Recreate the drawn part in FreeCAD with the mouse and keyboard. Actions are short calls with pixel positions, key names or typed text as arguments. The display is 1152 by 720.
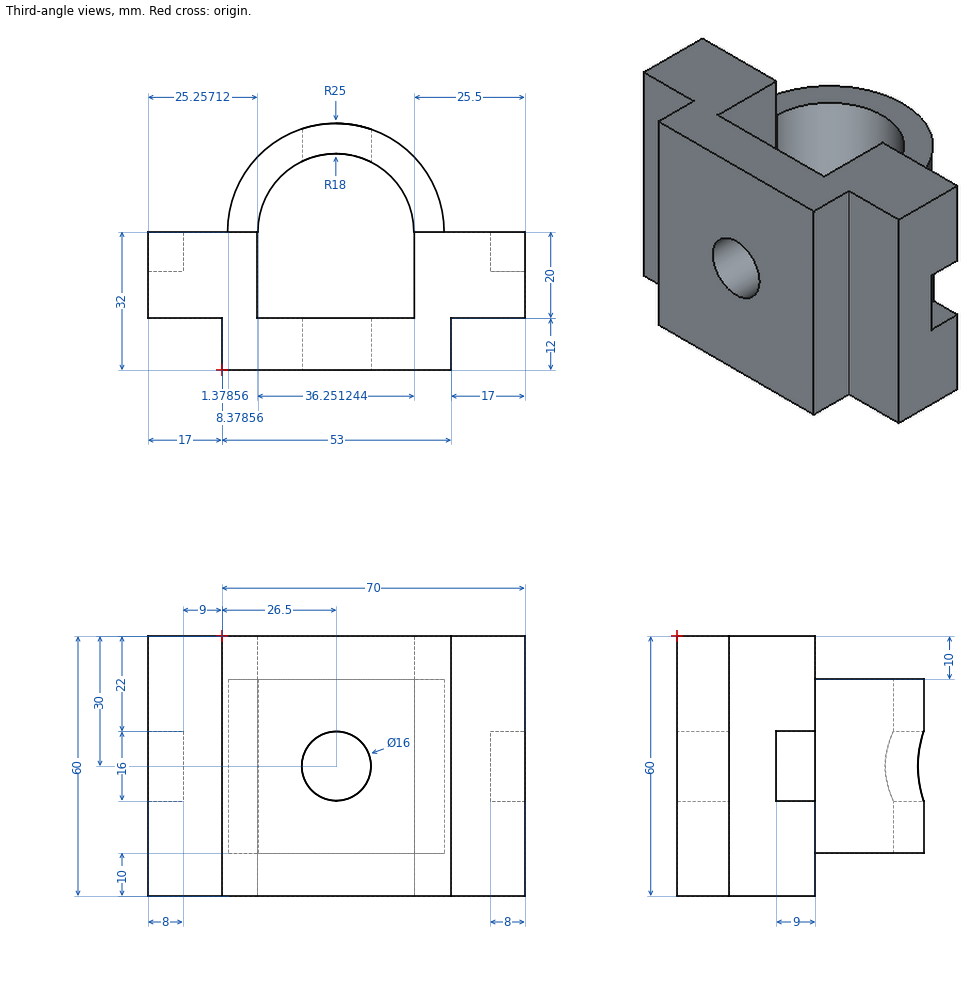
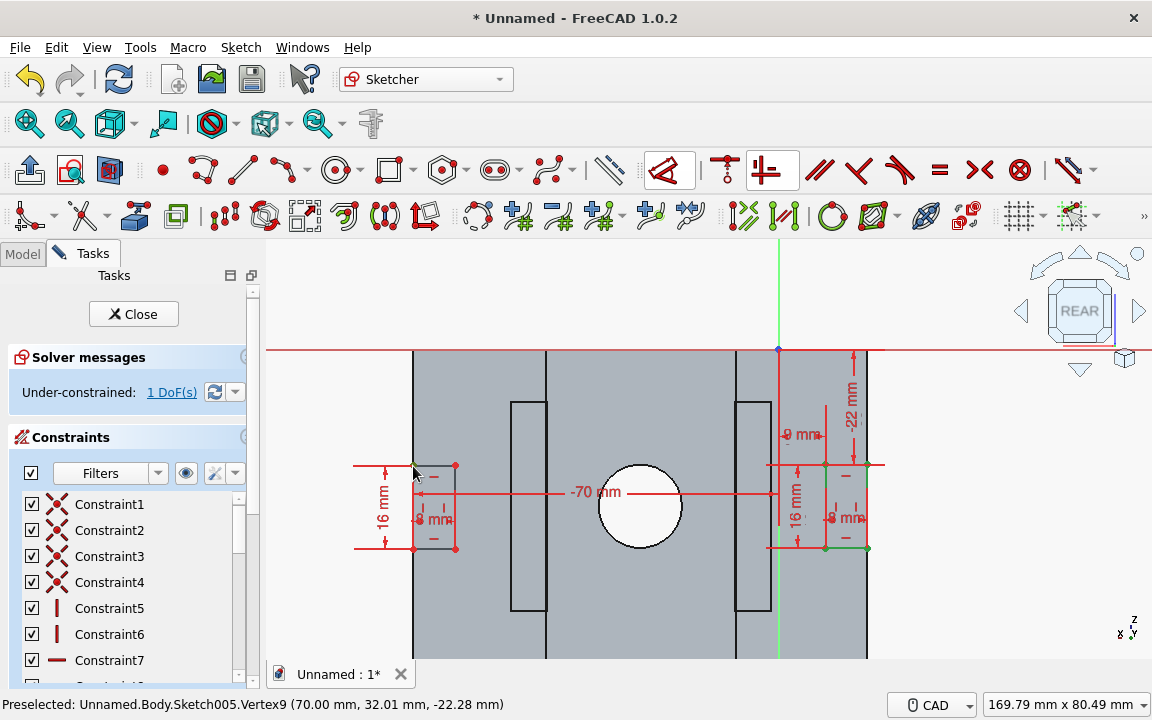
key(i)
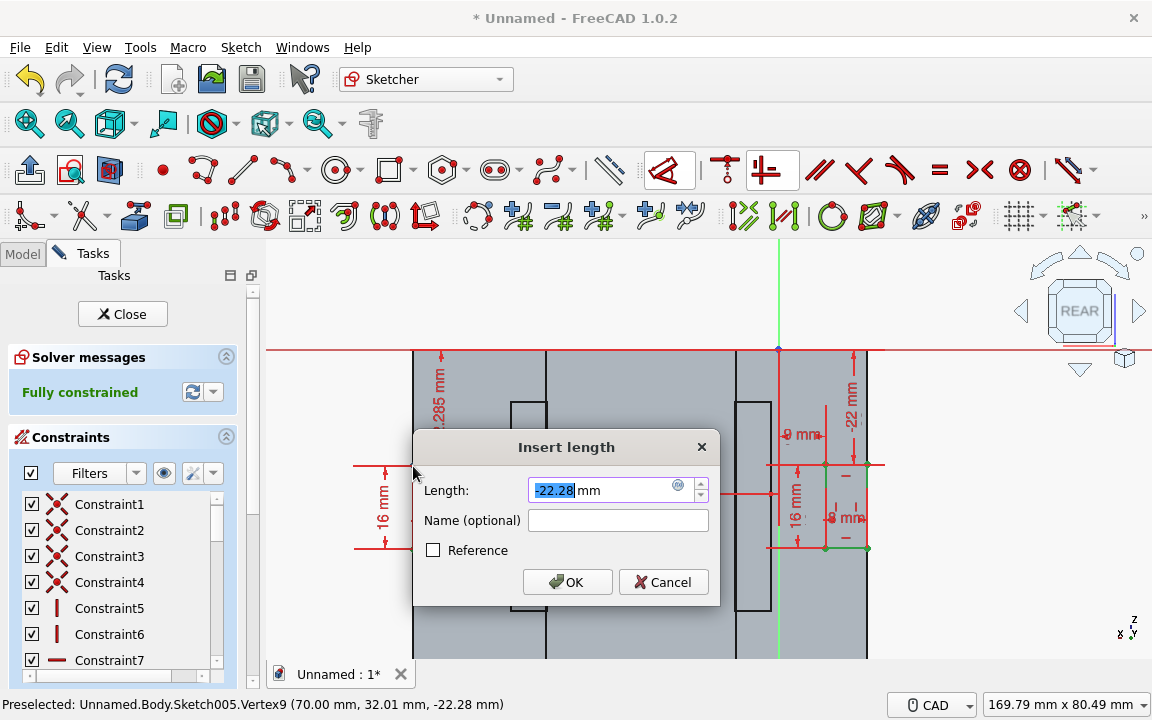
text(-22)
key(Return)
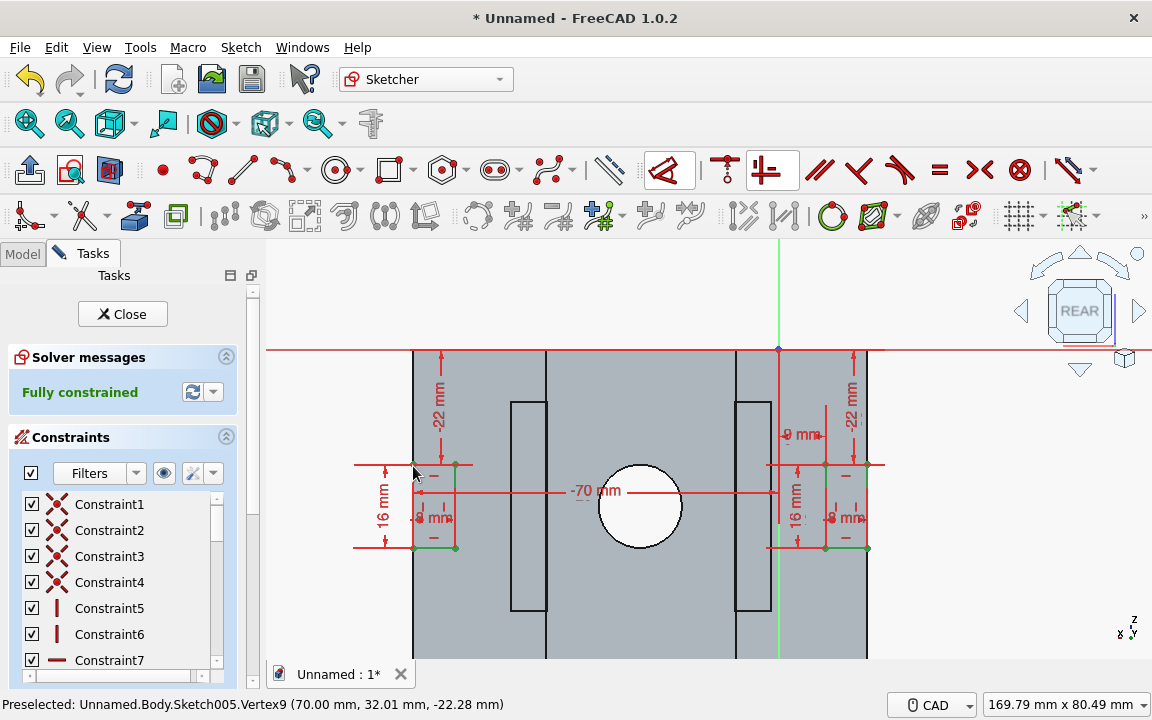
click(123, 314)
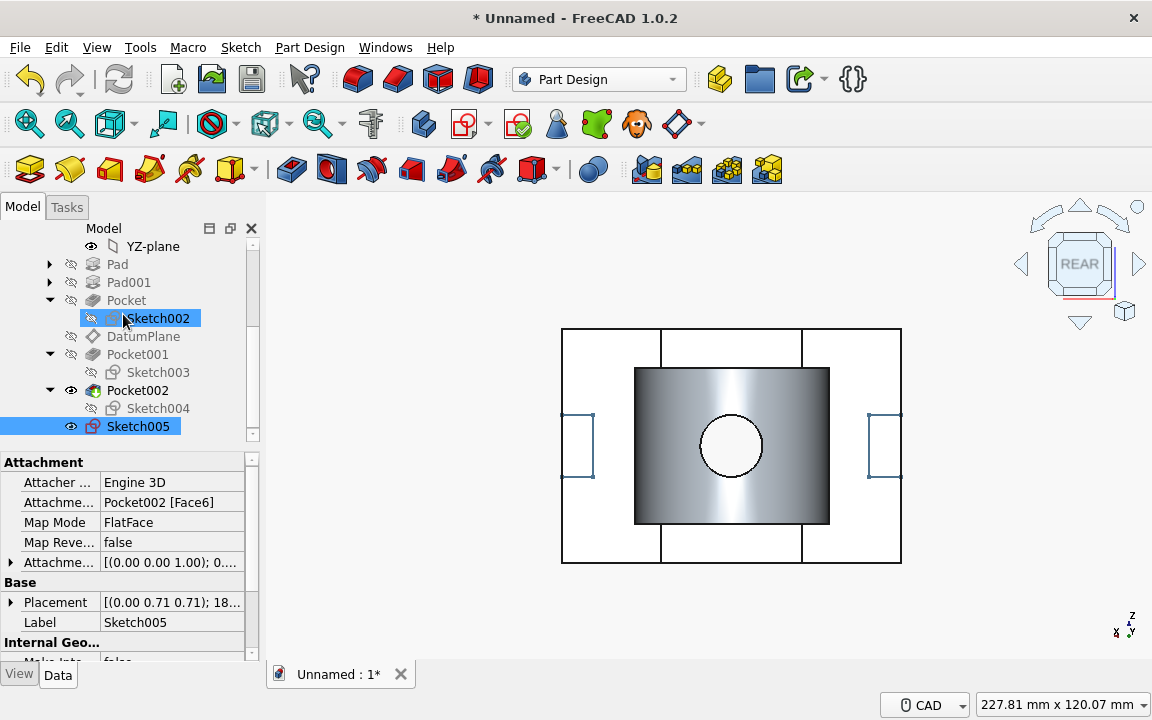
click(292, 170)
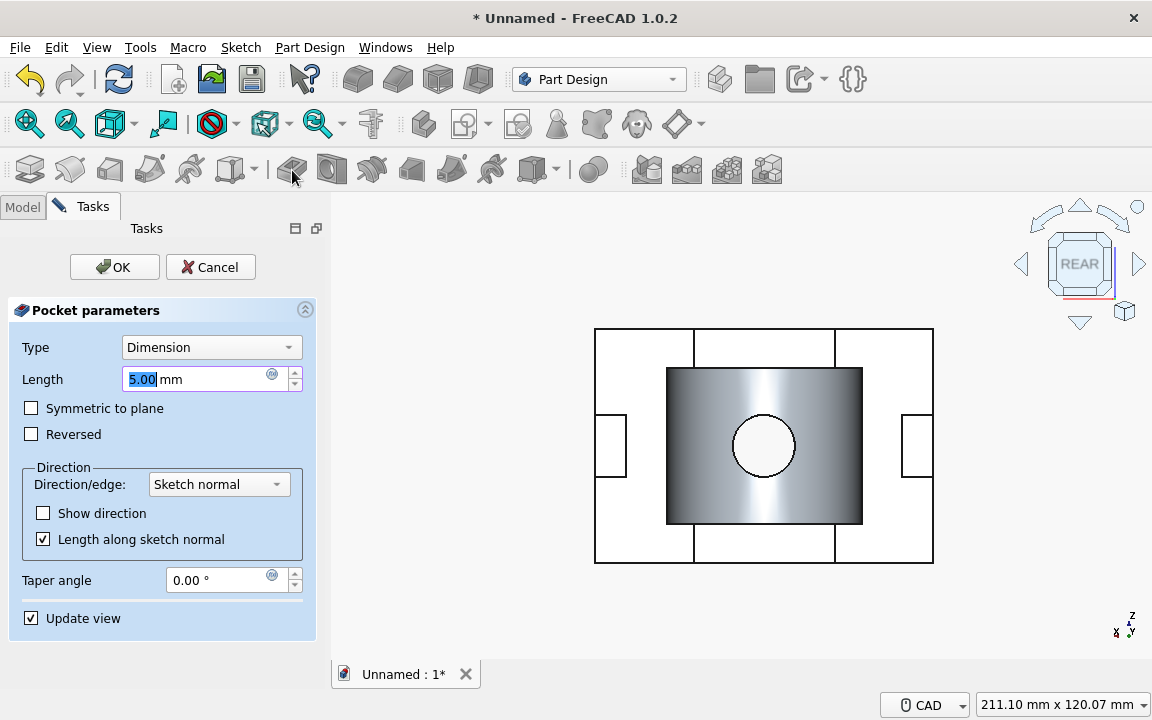
text(9)
key(Tab)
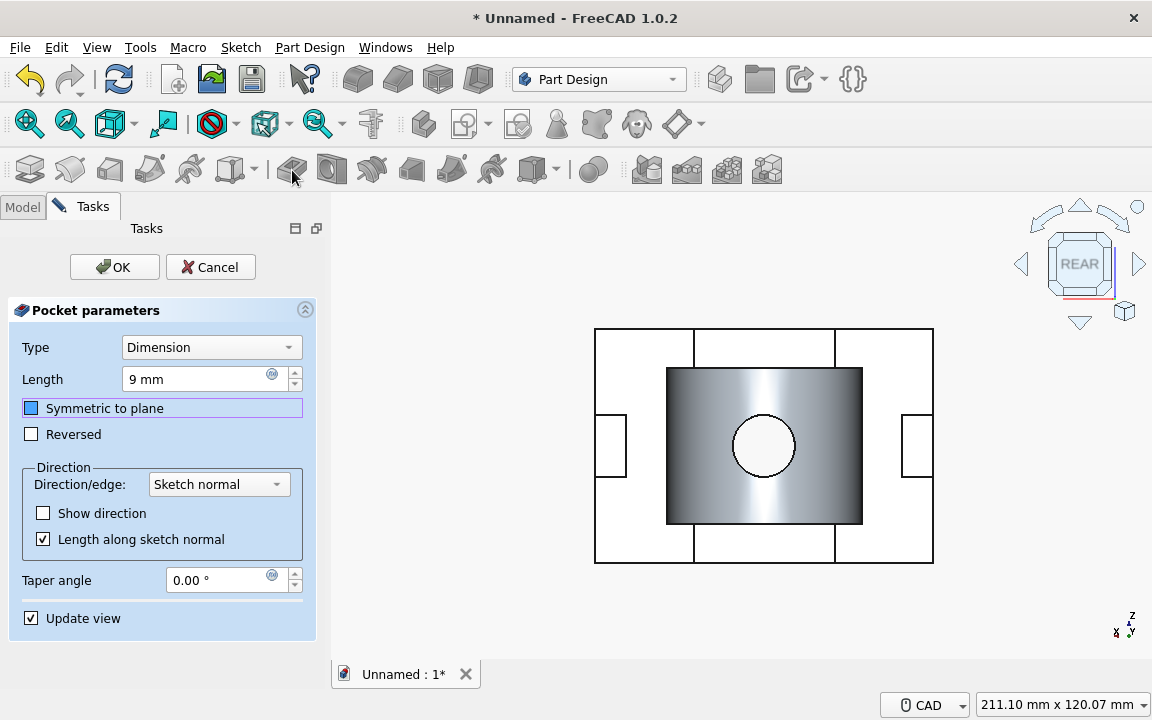
click(115, 267)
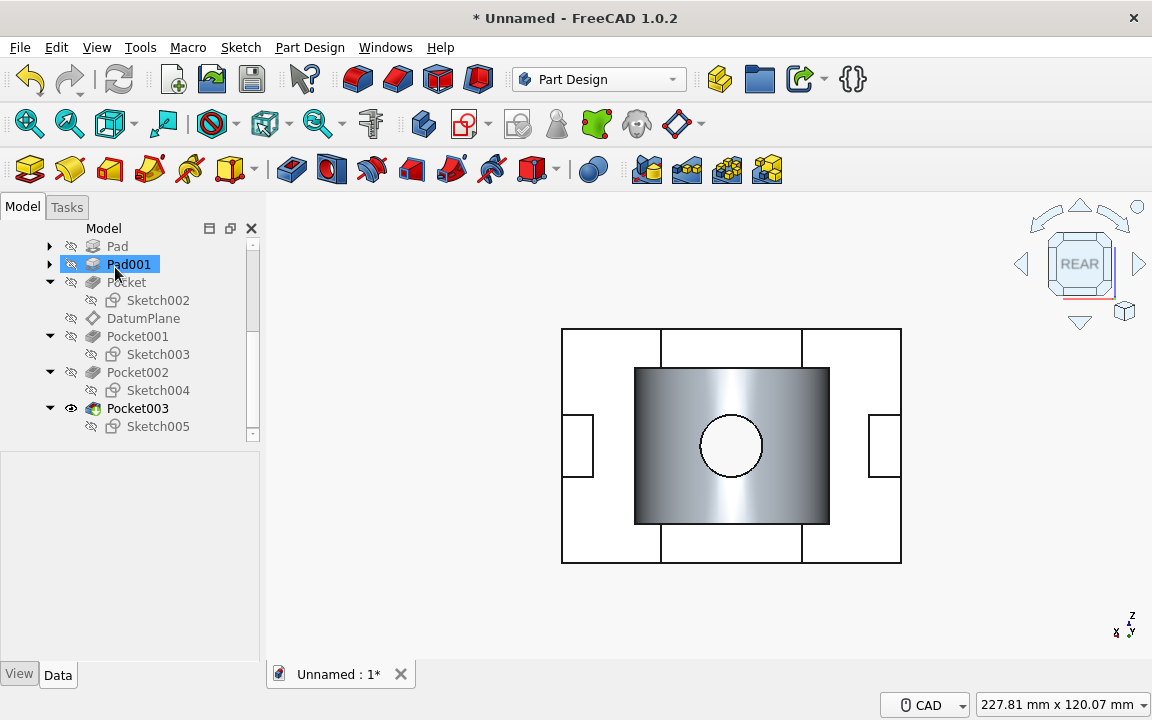
key(0)